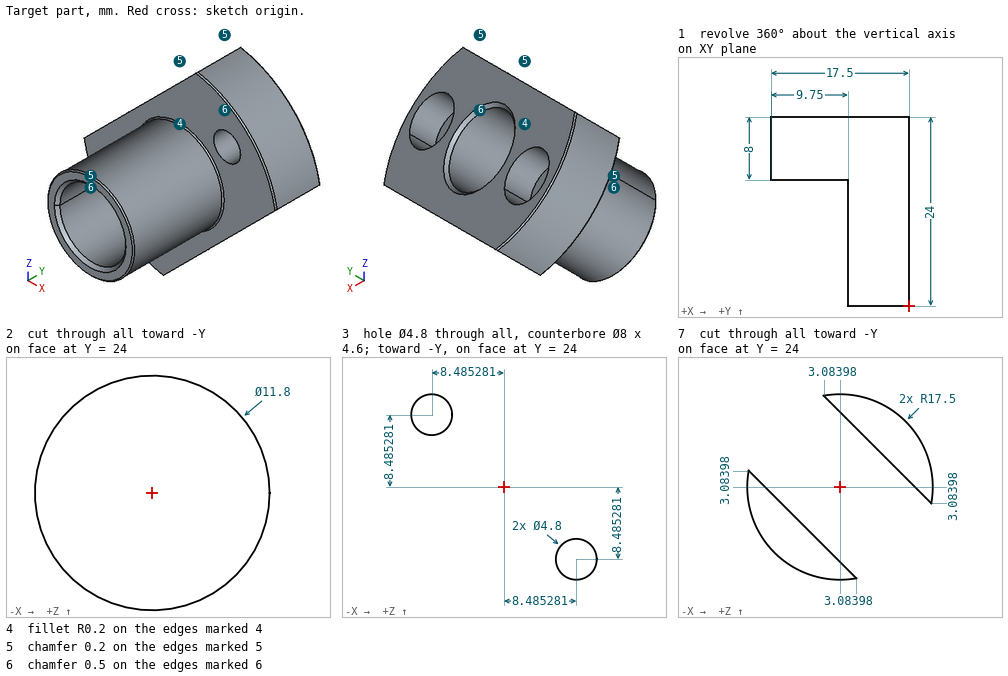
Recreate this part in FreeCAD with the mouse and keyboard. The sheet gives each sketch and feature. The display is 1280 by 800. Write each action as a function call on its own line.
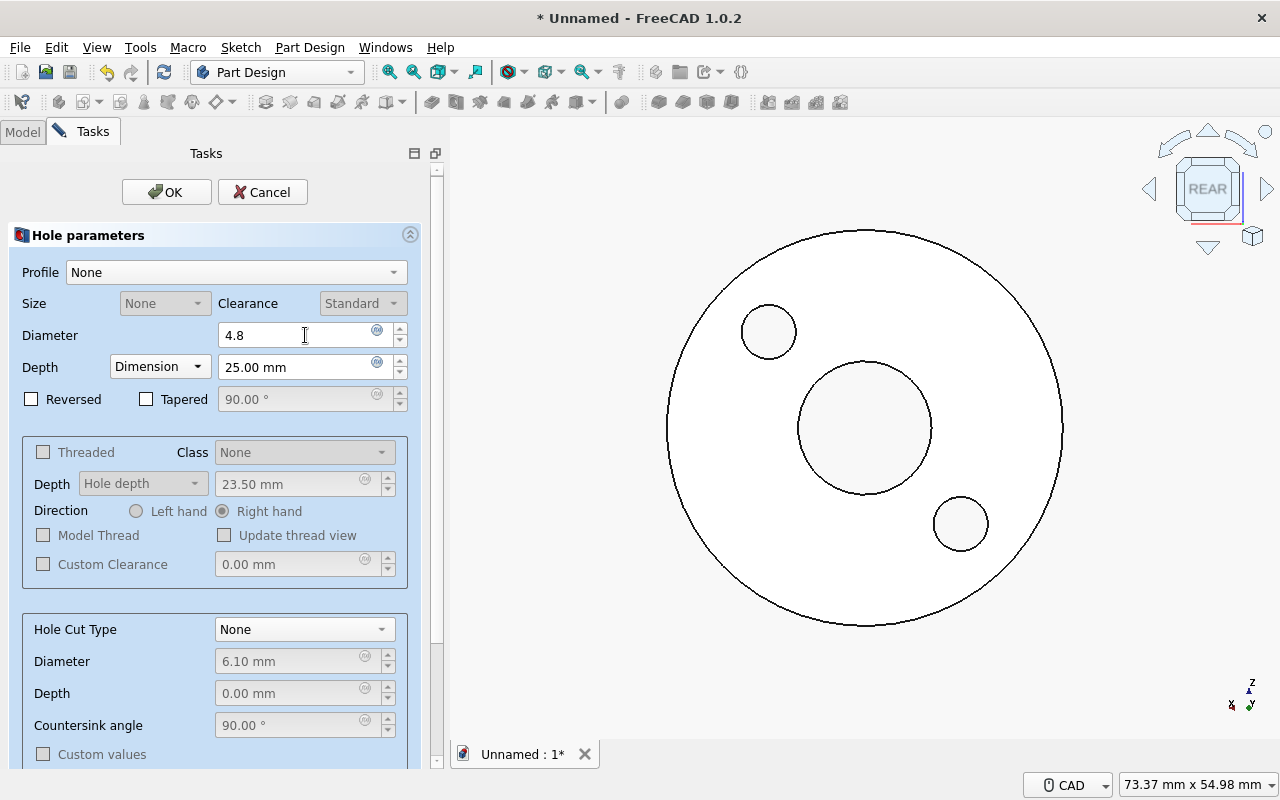
click(161, 366)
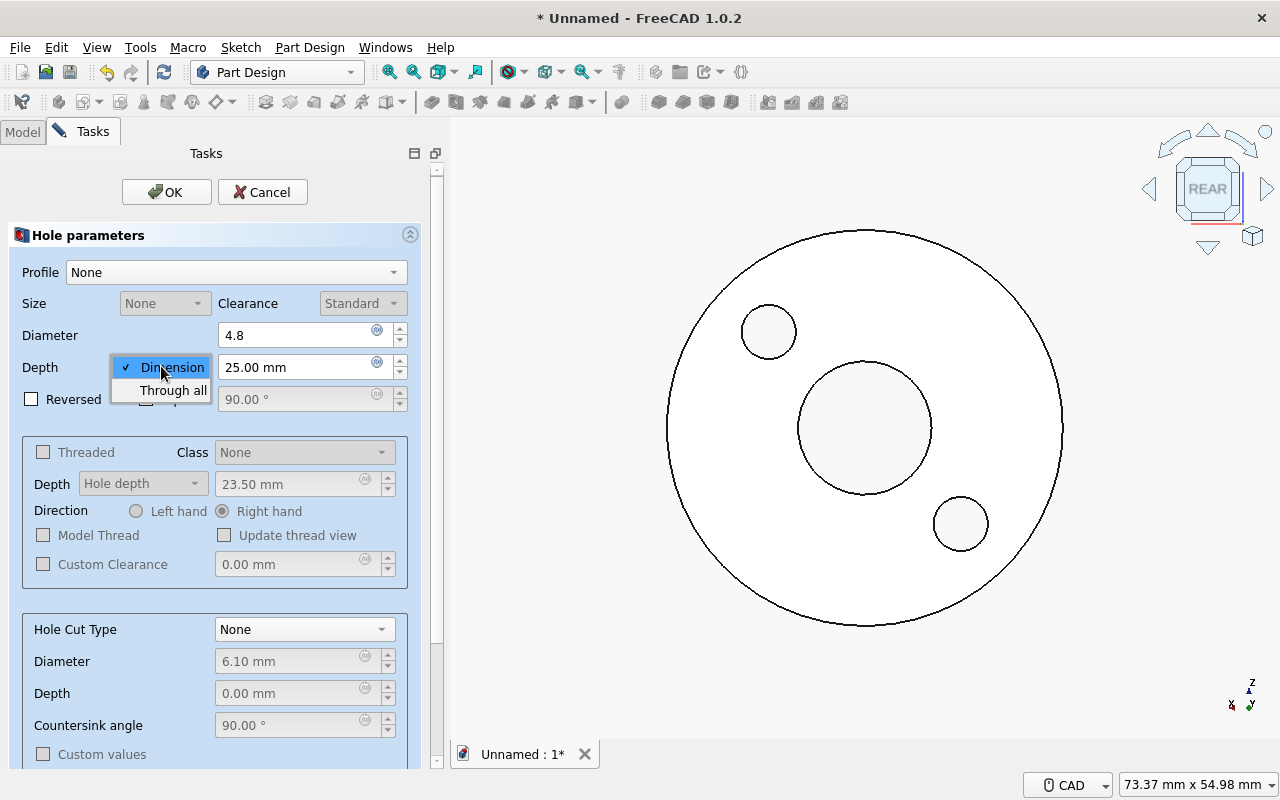
click(160, 390)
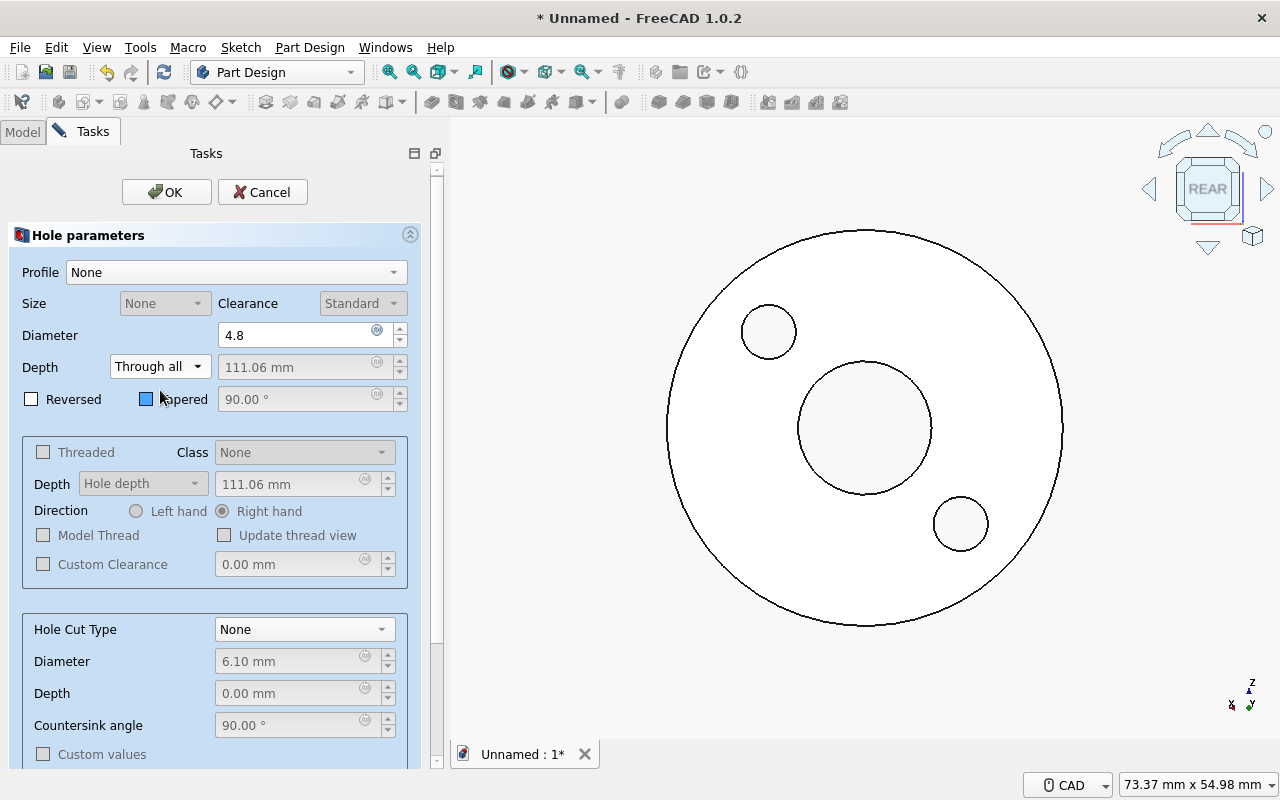
click(306, 630)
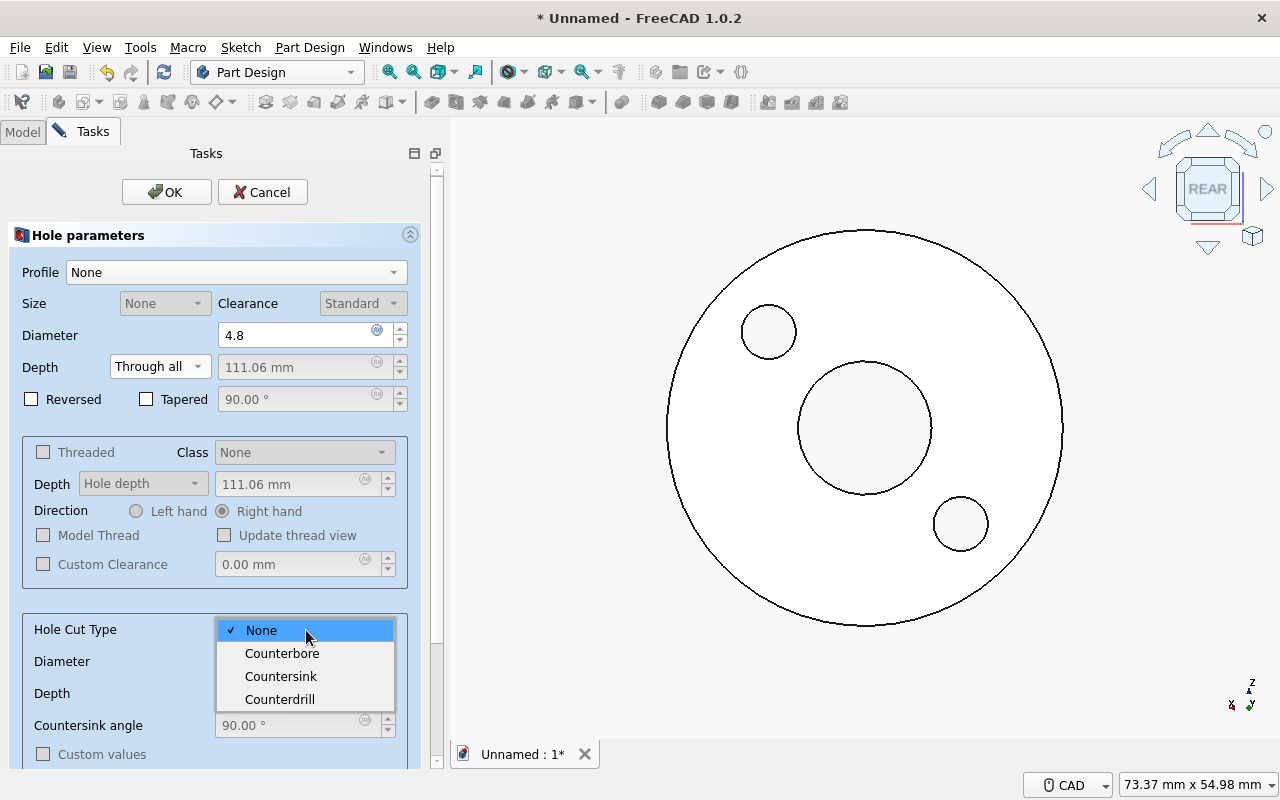
click(304, 654)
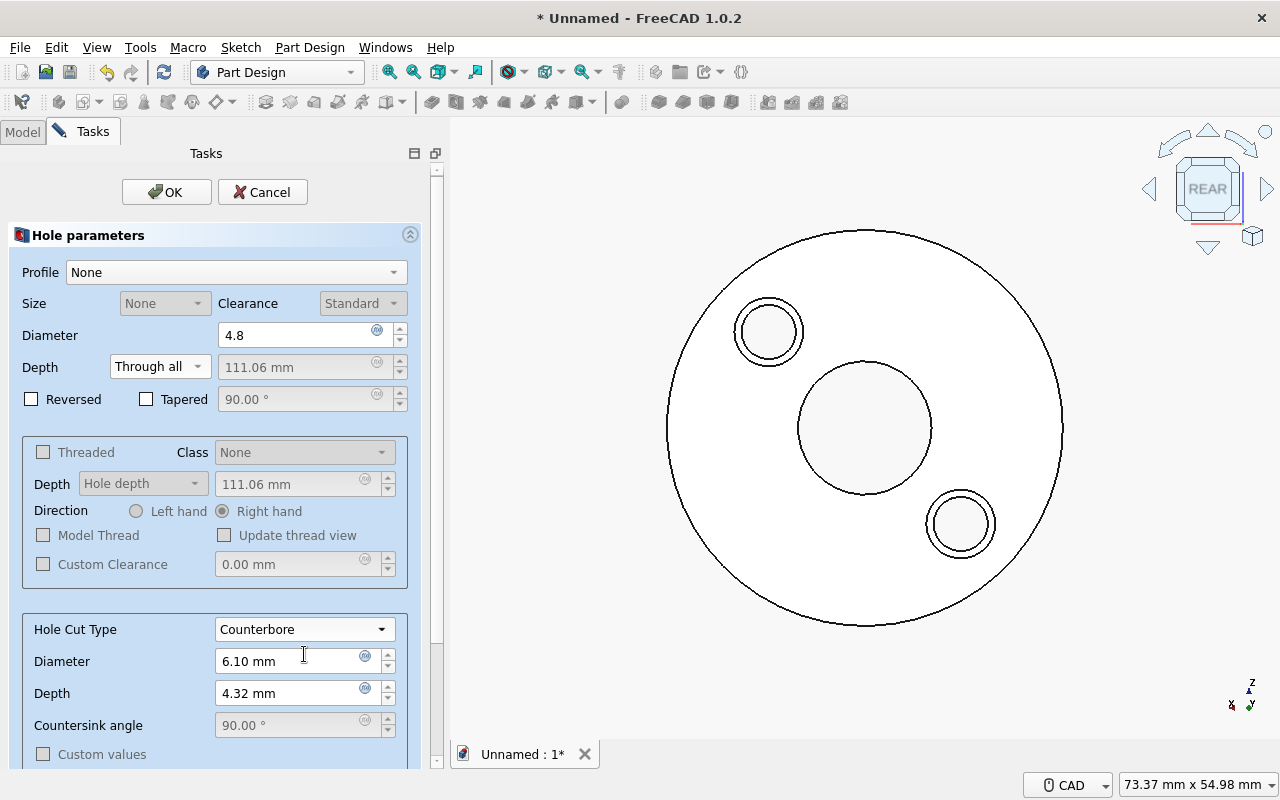
triple_click(298, 661)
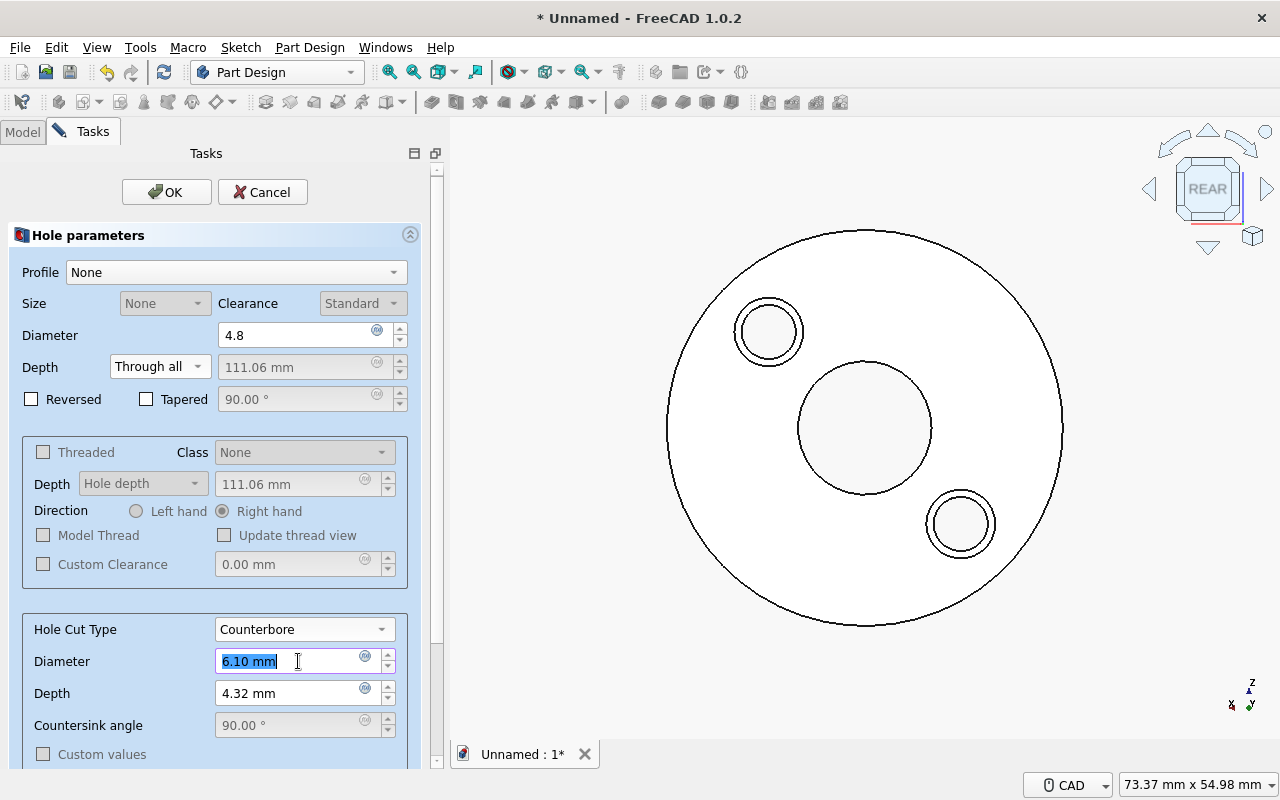
text(8)
key(Tab)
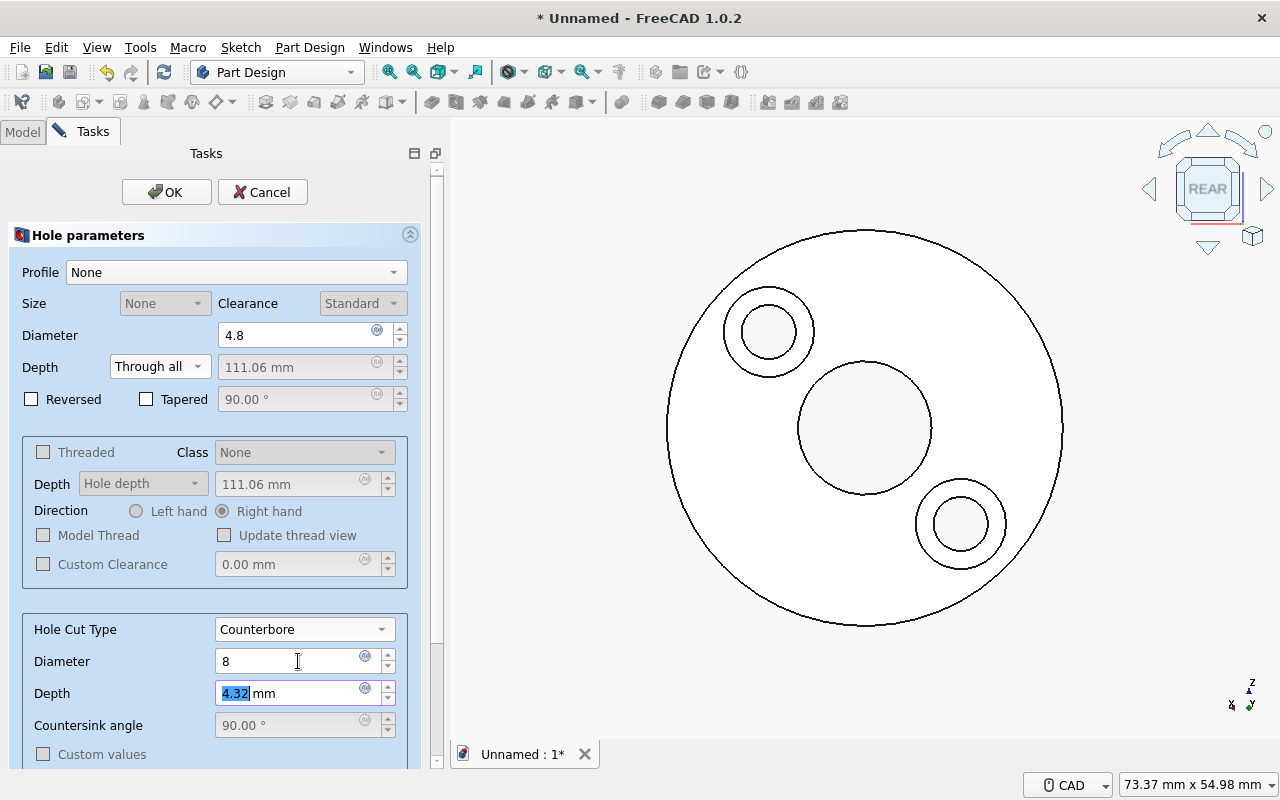
text(4.6)
key(Tab)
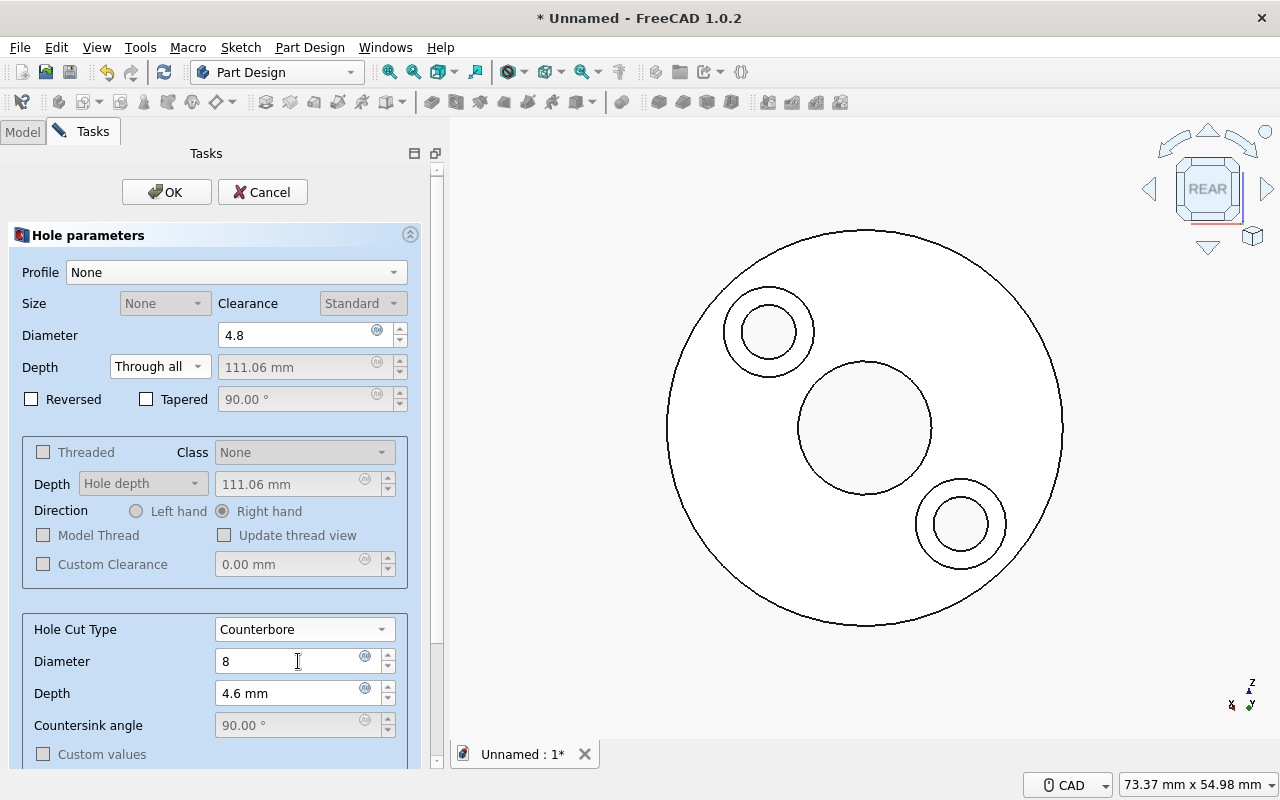
click(167, 192)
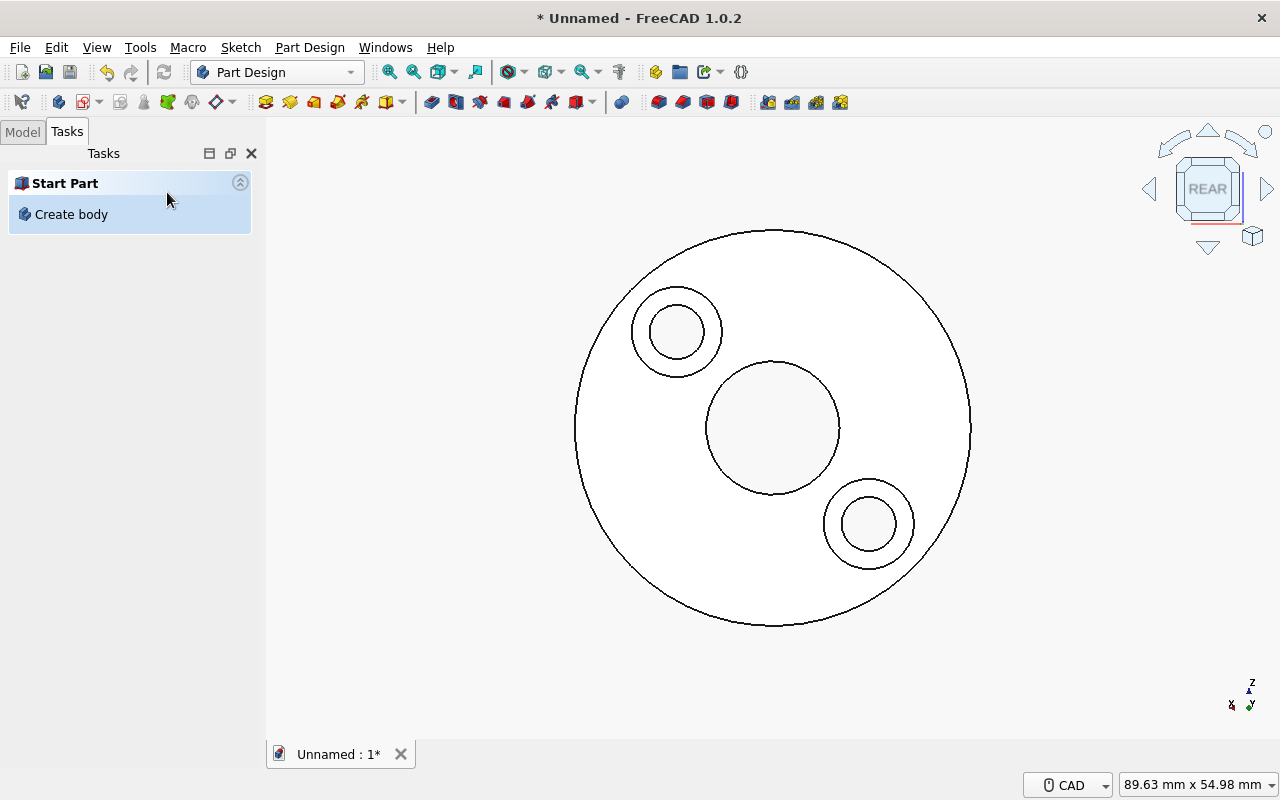
key(0)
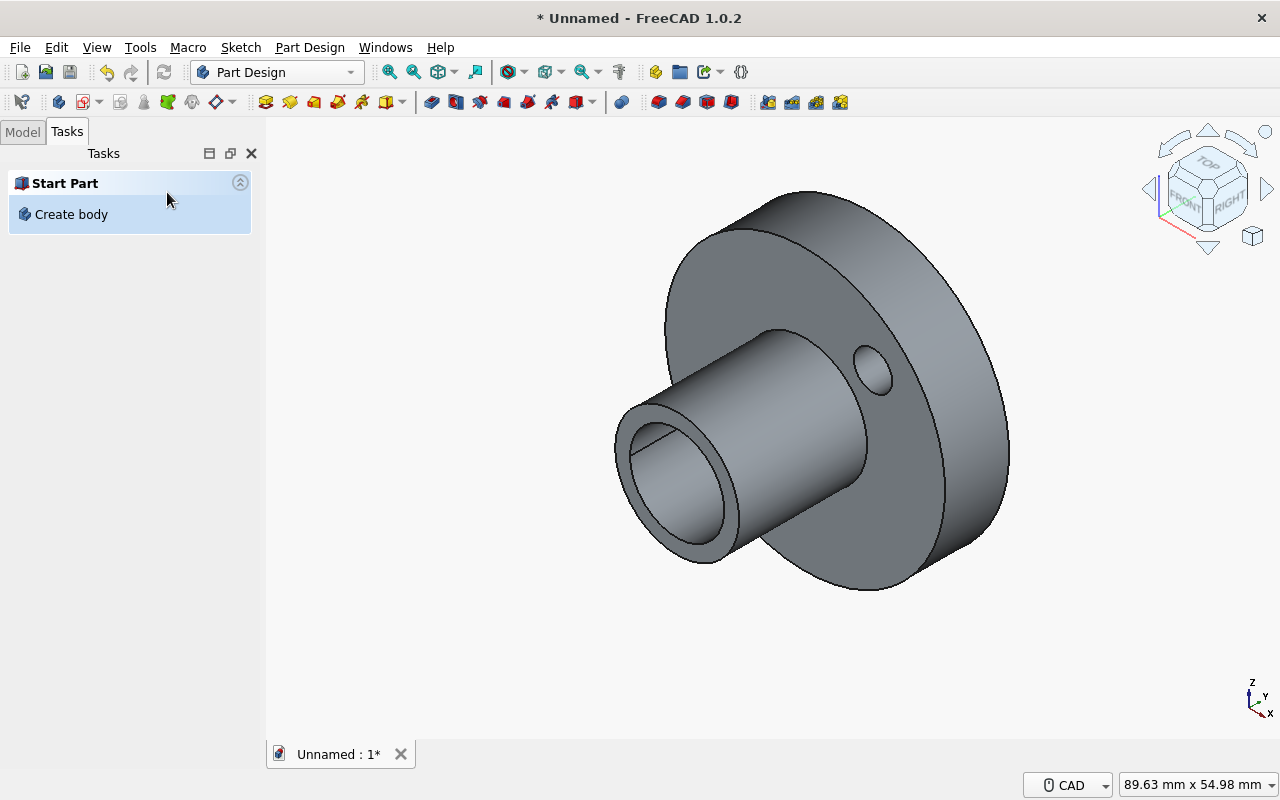
key(2)